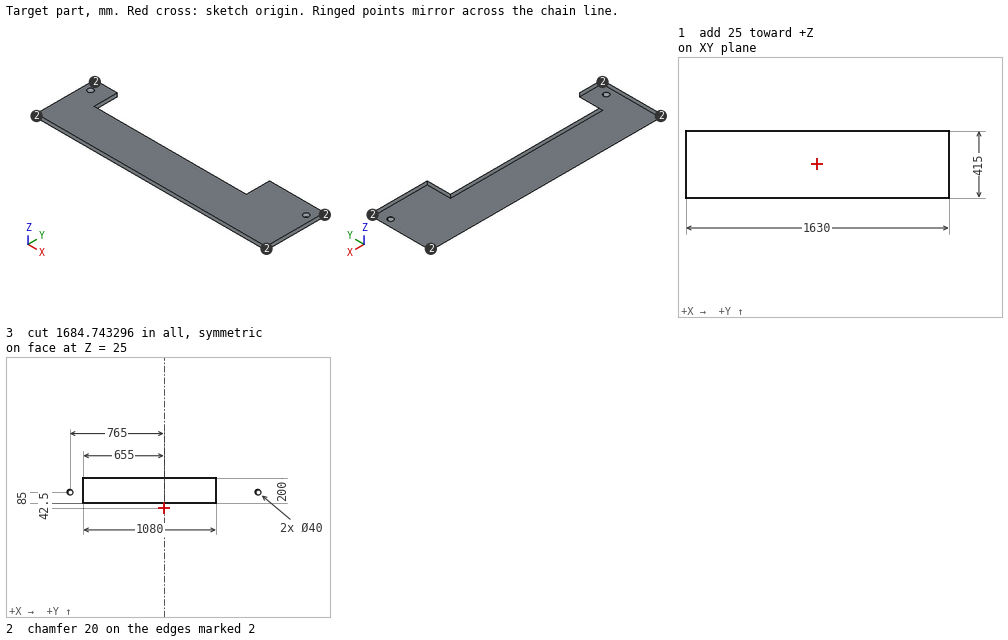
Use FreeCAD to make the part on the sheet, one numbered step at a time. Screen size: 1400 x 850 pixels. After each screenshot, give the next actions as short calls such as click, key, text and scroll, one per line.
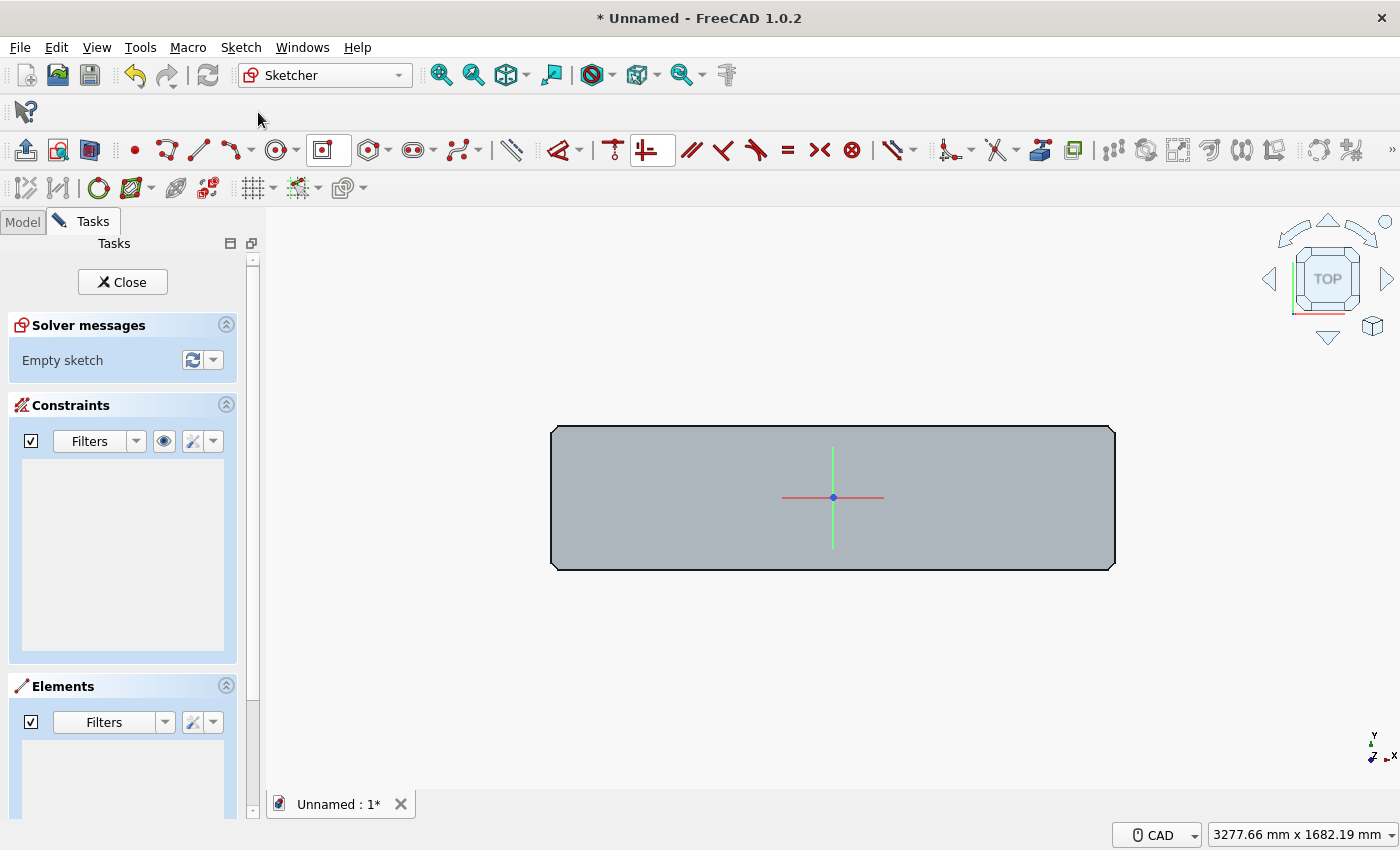
click(346, 150)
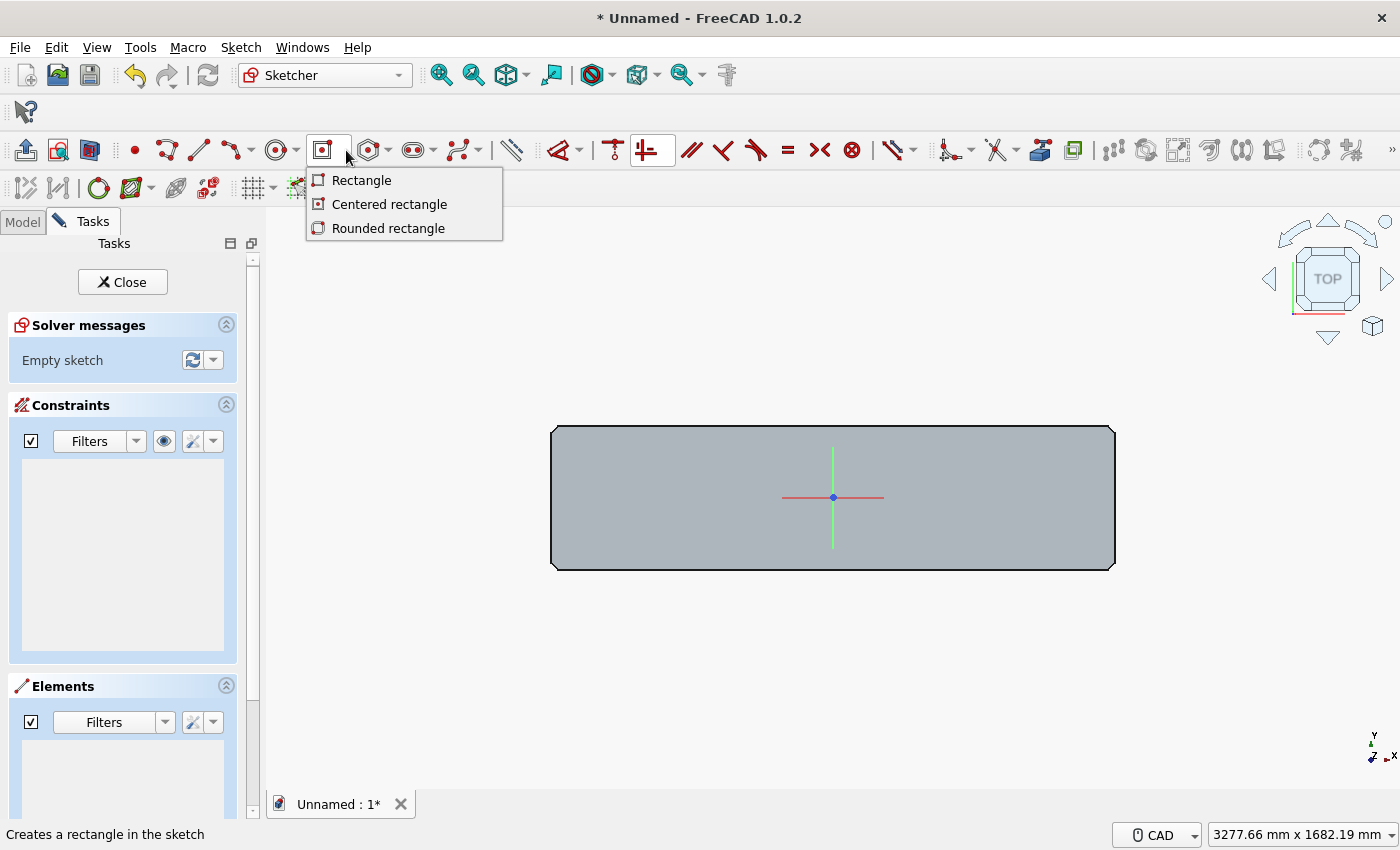
click(404, 180)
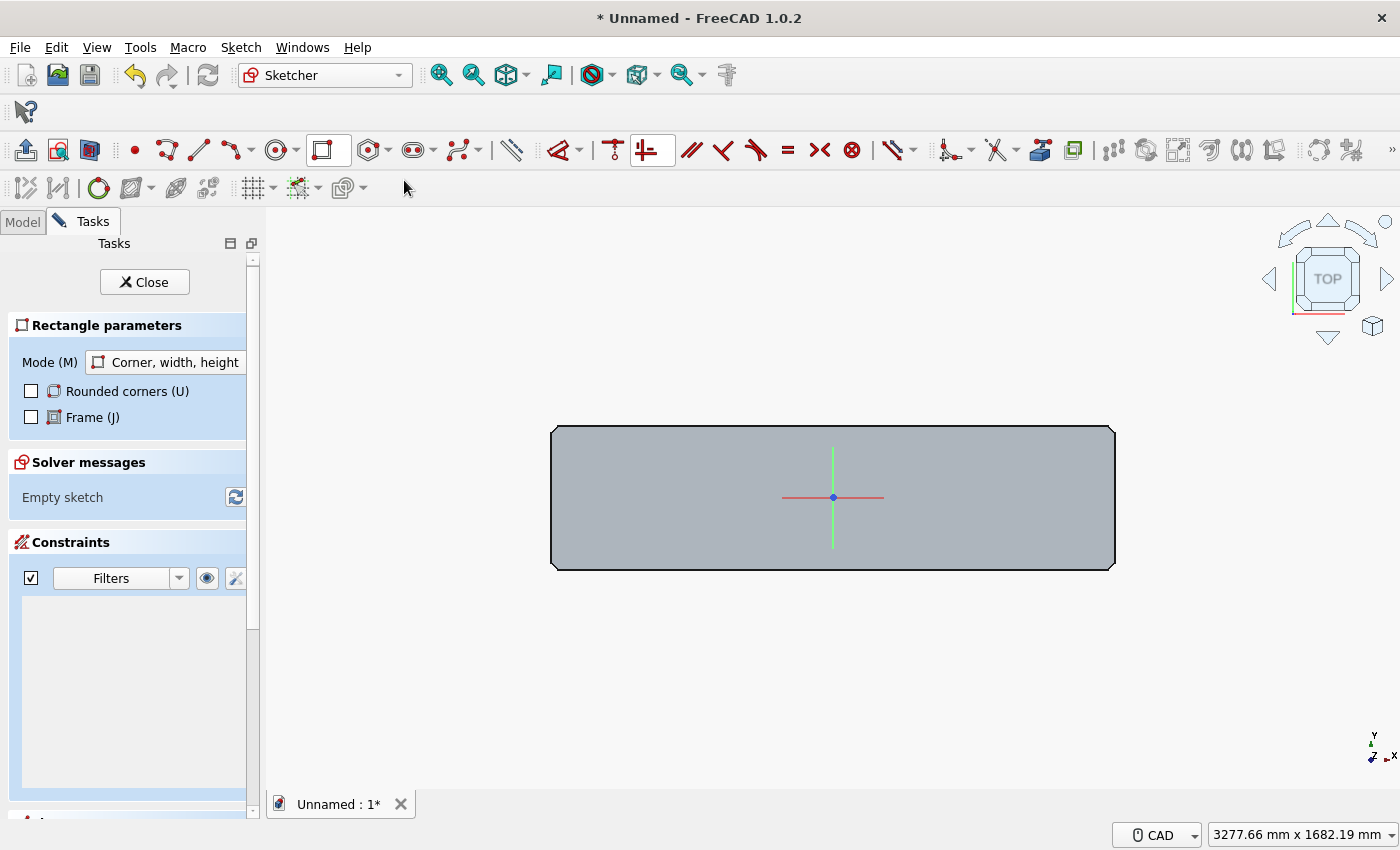
click(606, 414)
move(980, 483)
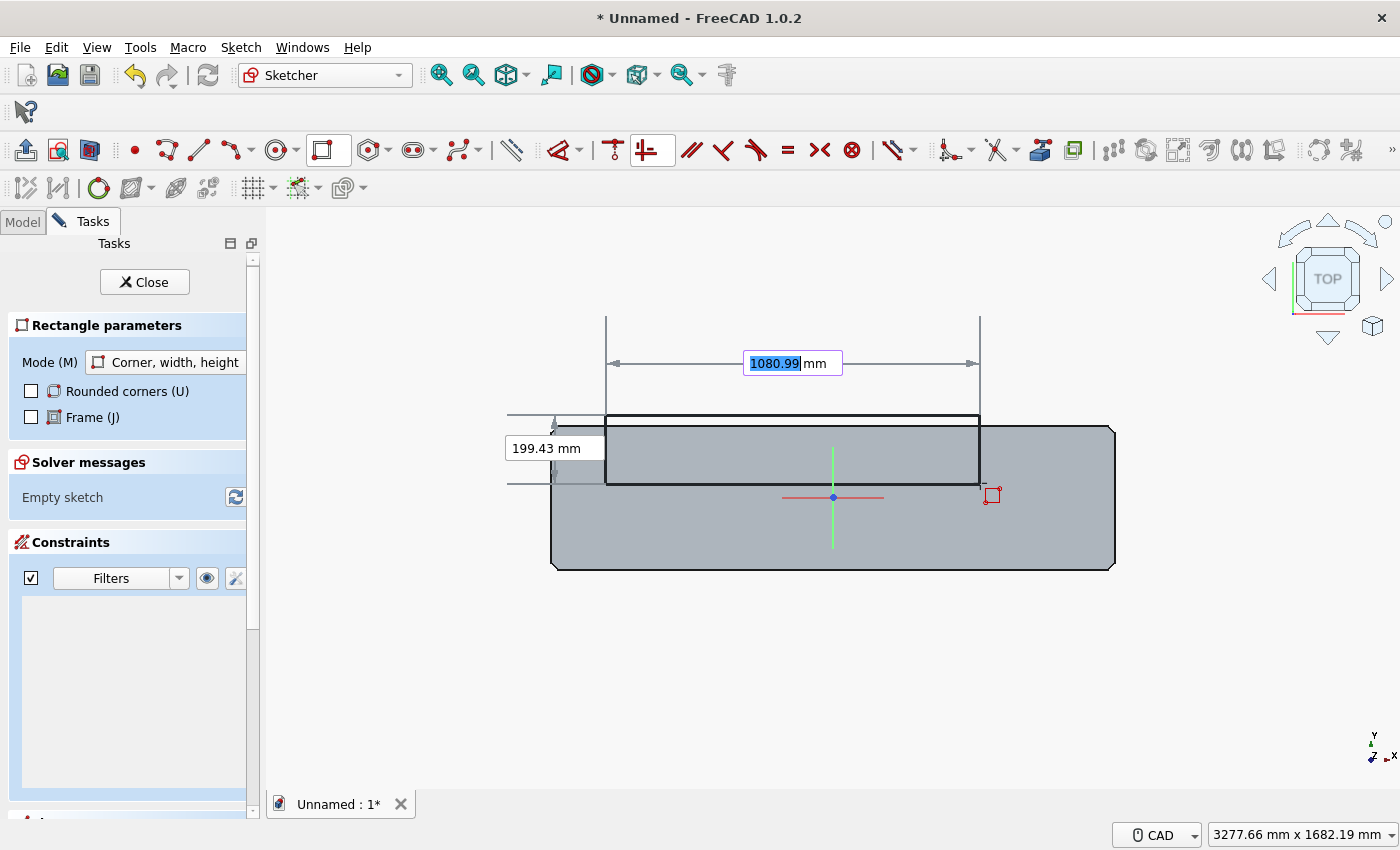
text(1080)
key(Tab)
text(200)
key(Return)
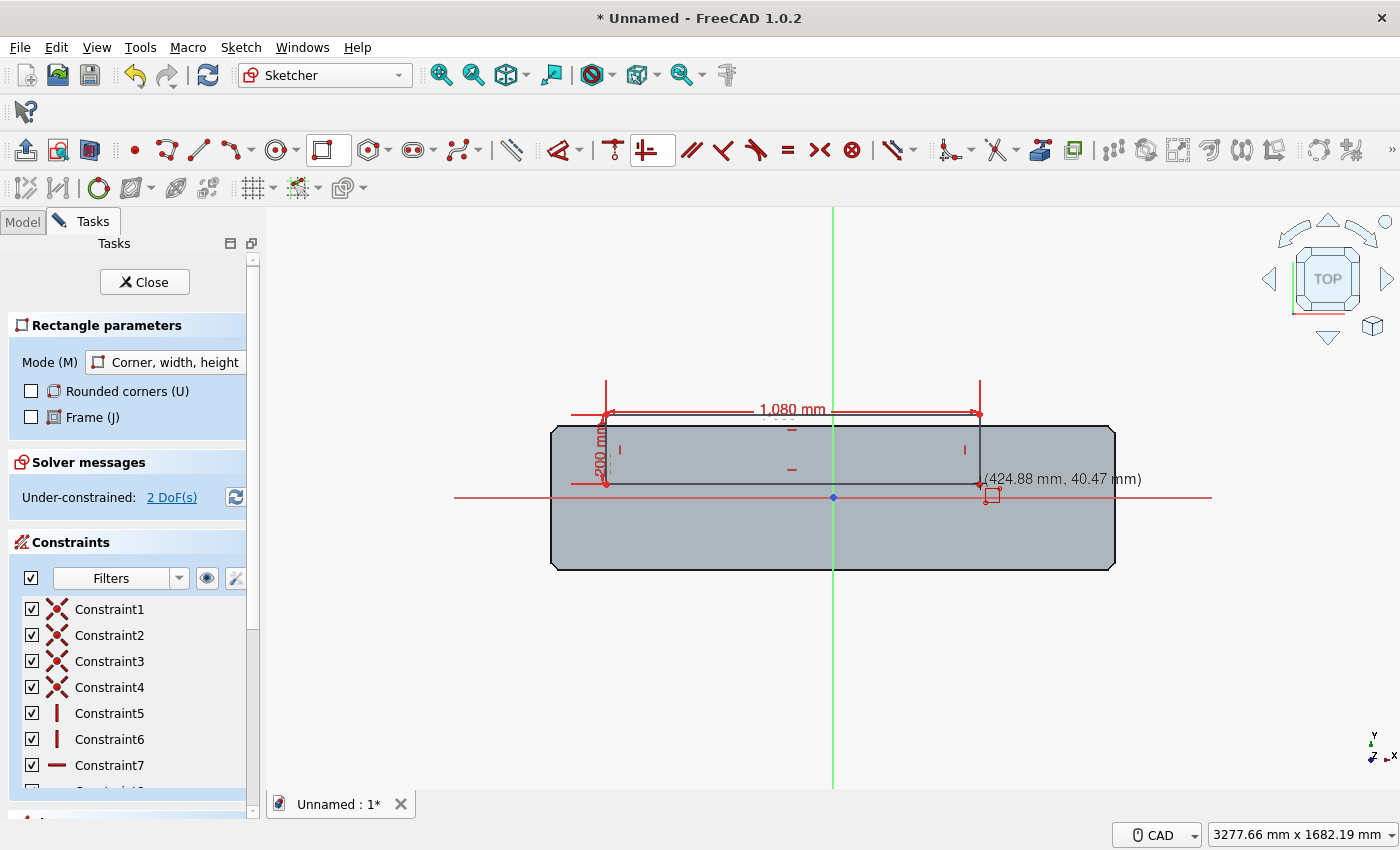
click(276, 150)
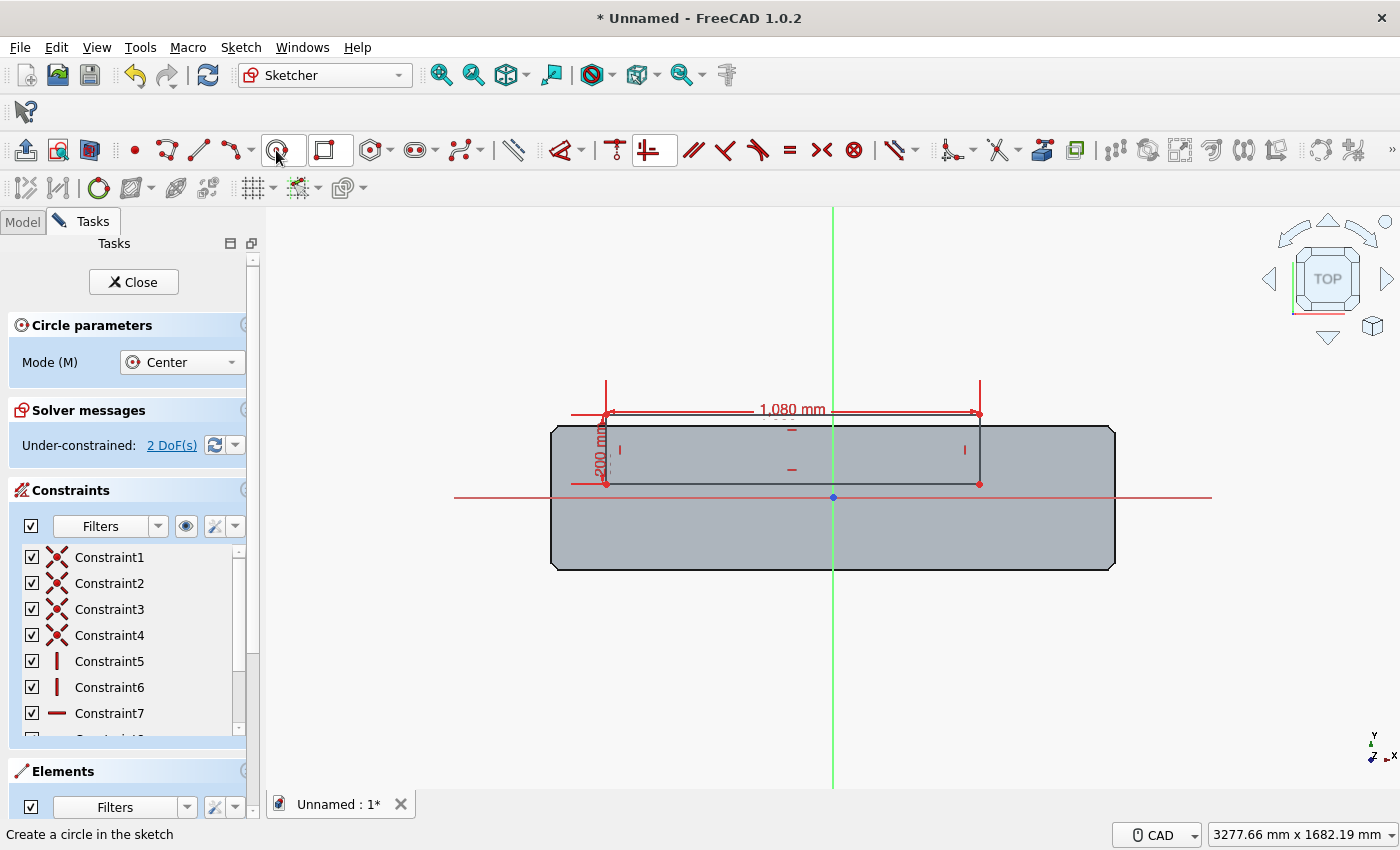
scroll(568, 454, up, 6)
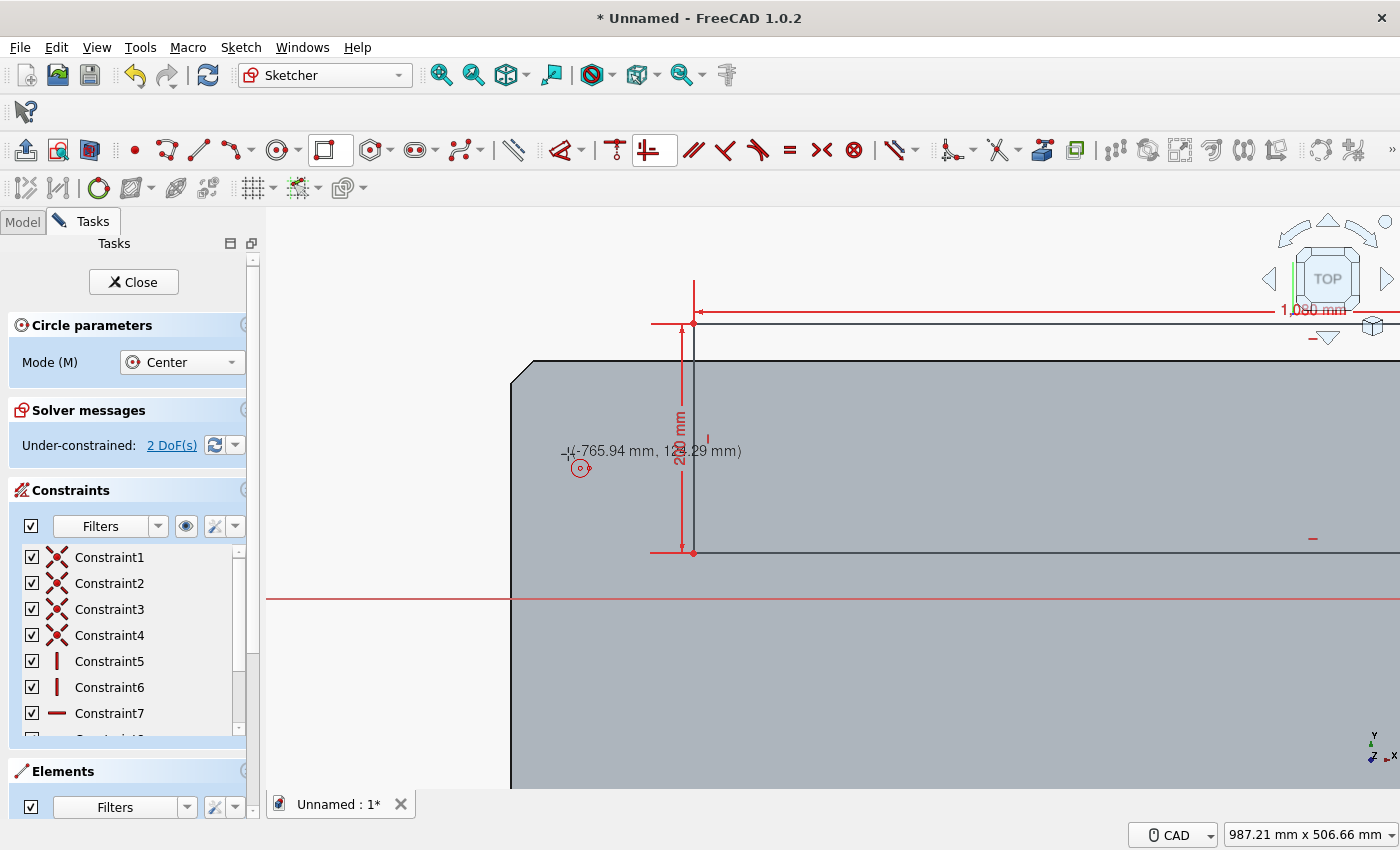
click(568, 453)
move(585, 436)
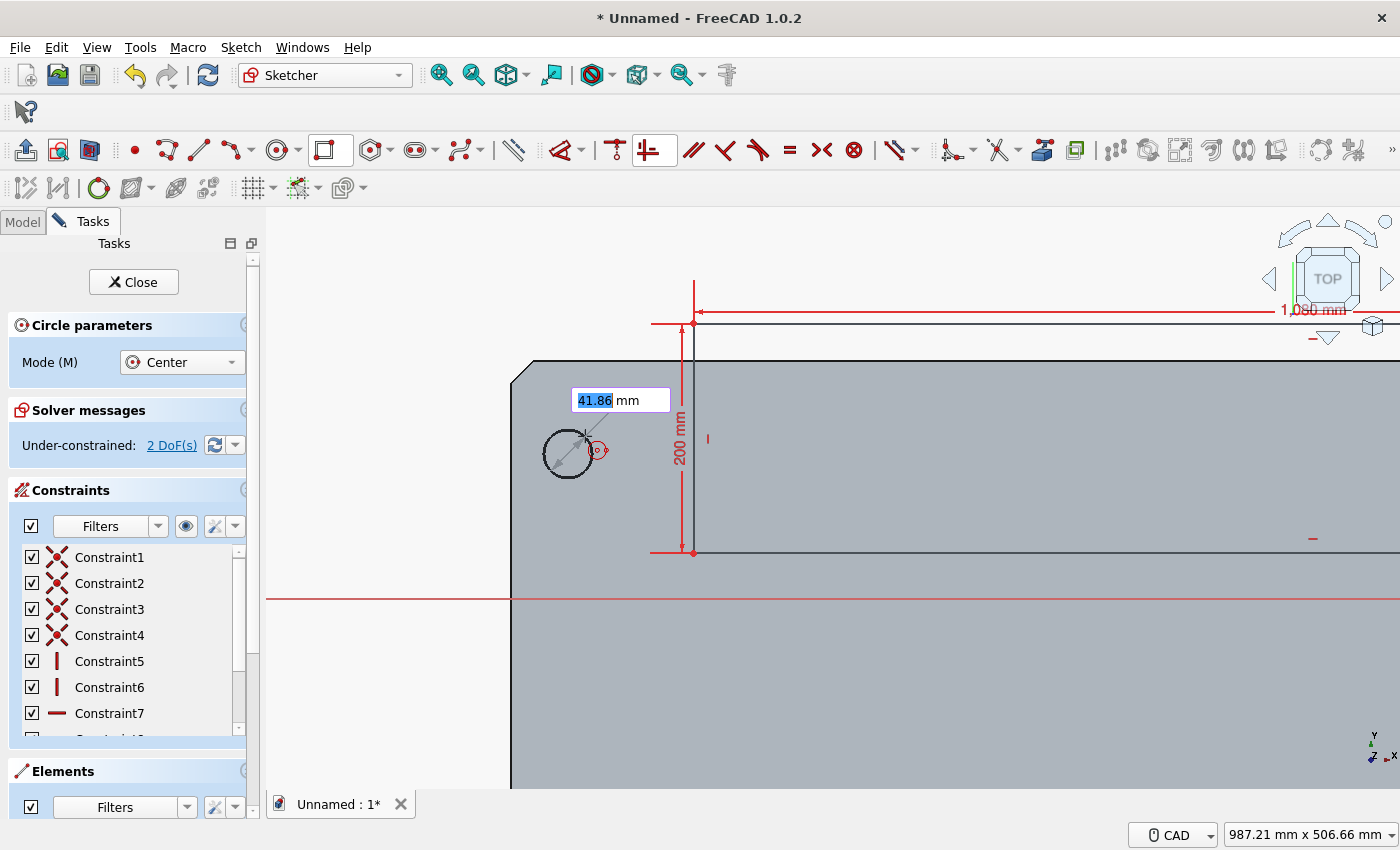
text(40)
key(Return)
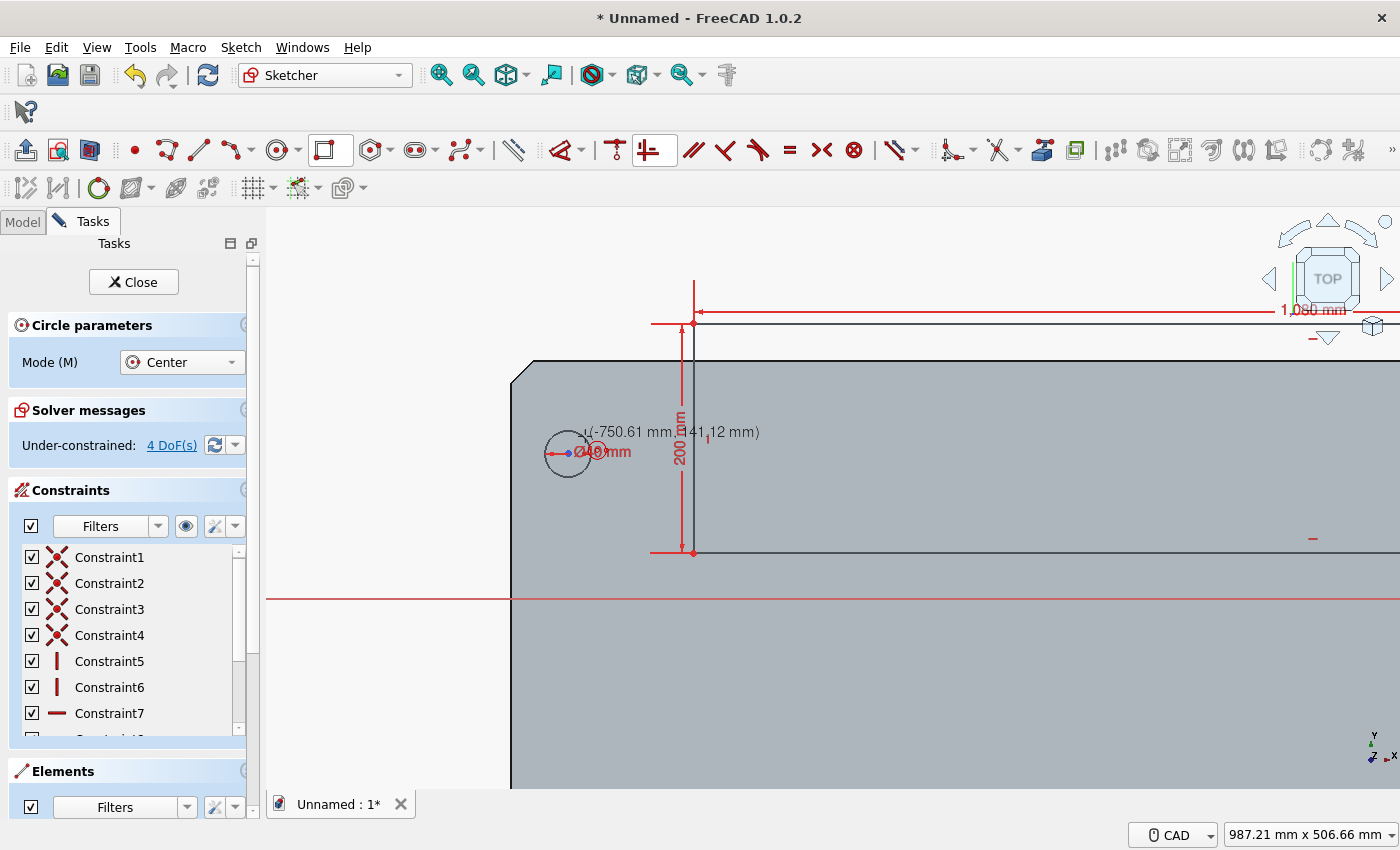
scroll(367, 520, down, 5)